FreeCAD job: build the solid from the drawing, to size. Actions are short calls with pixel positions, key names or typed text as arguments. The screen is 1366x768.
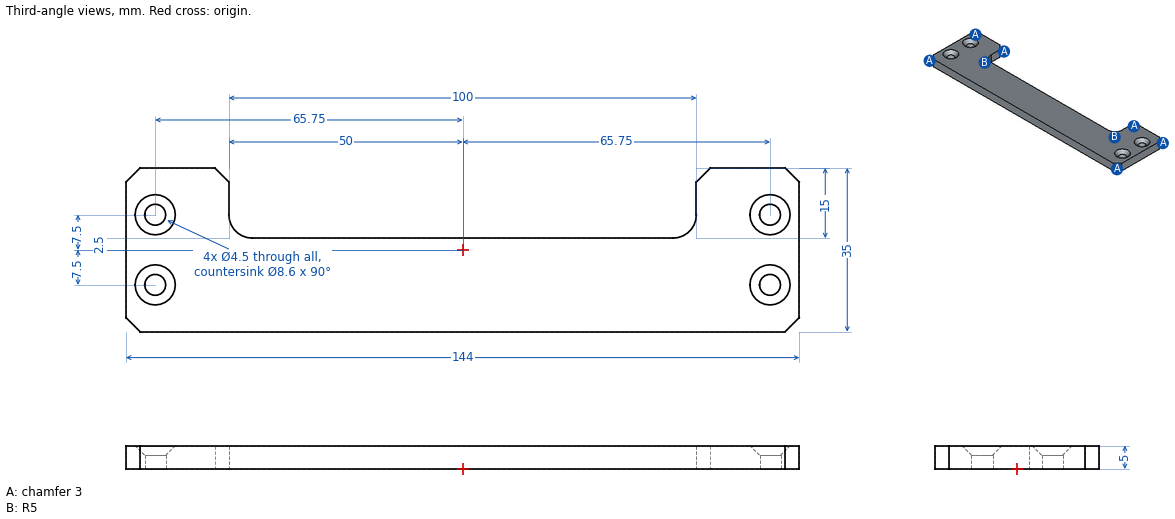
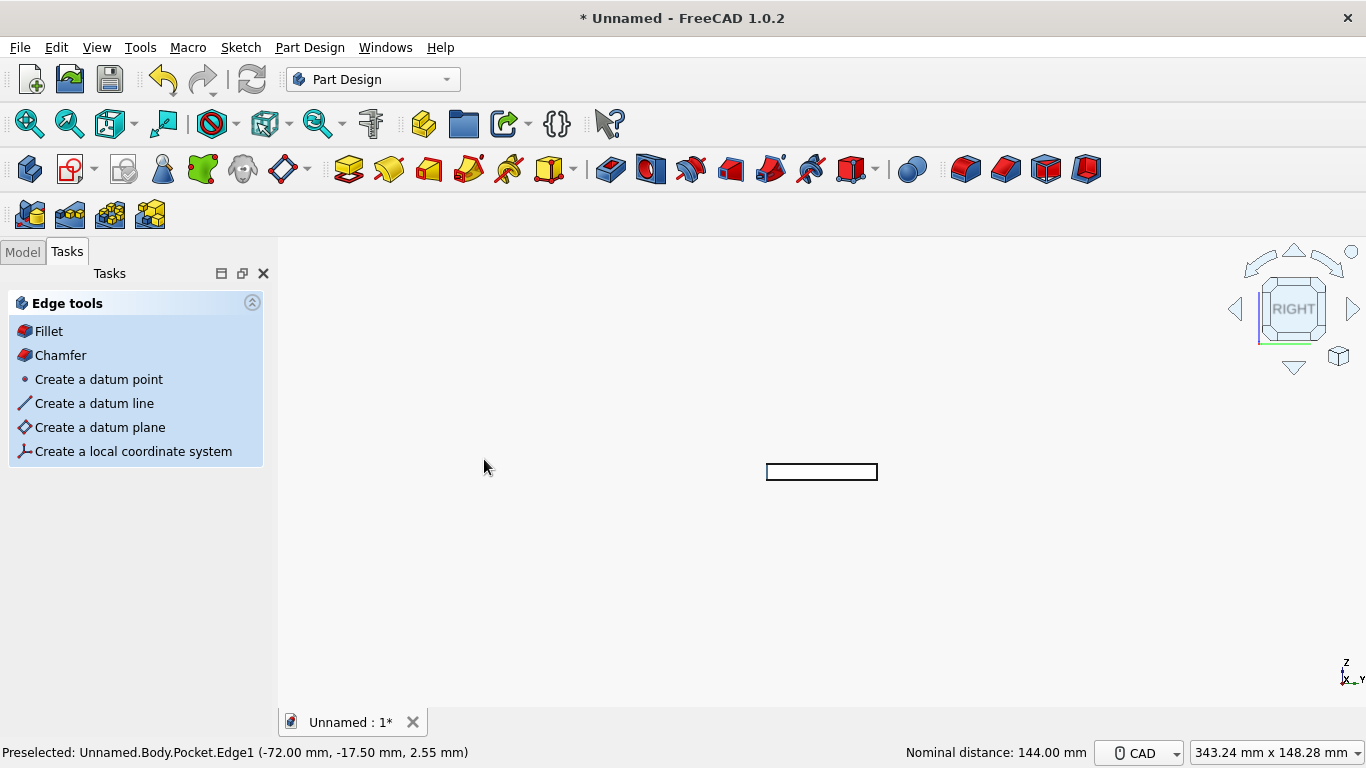
click(877, 471, ctrl)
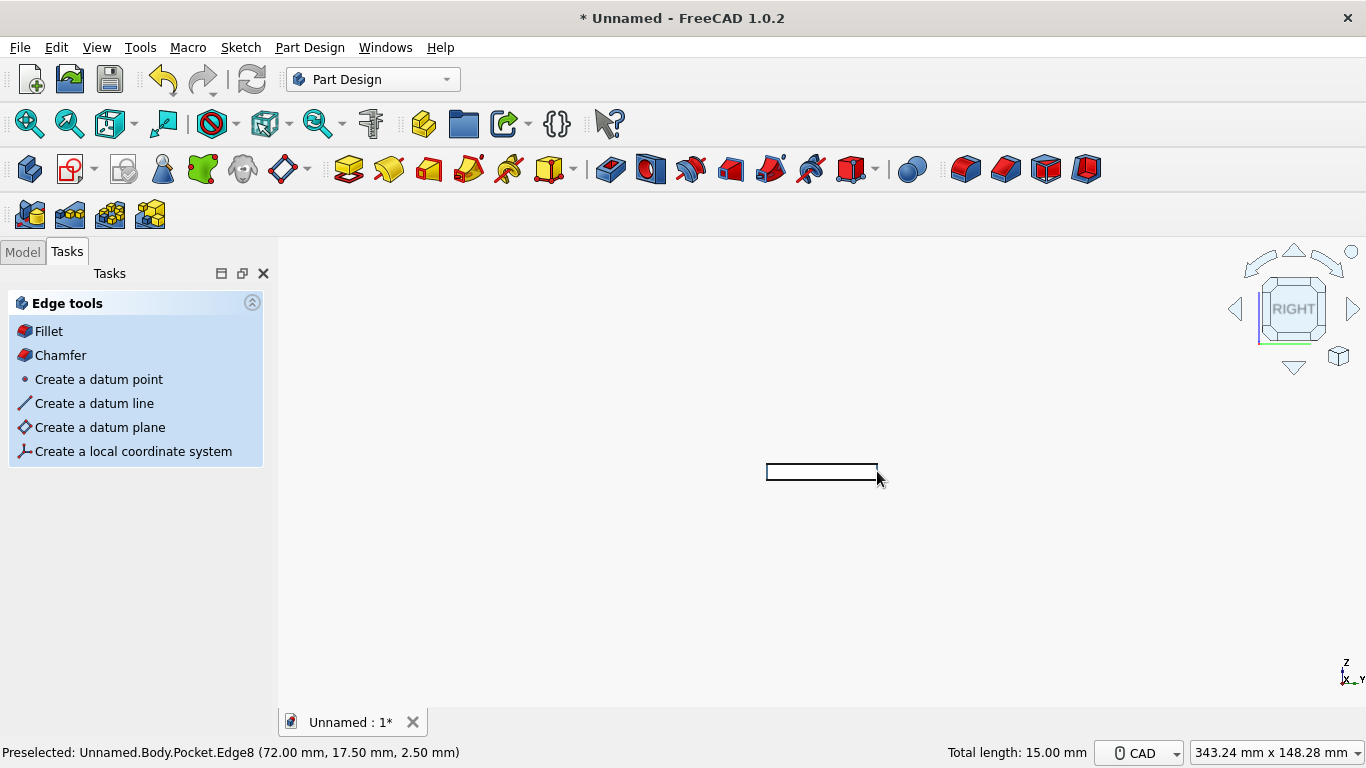
scroll(877, 471, up, 5)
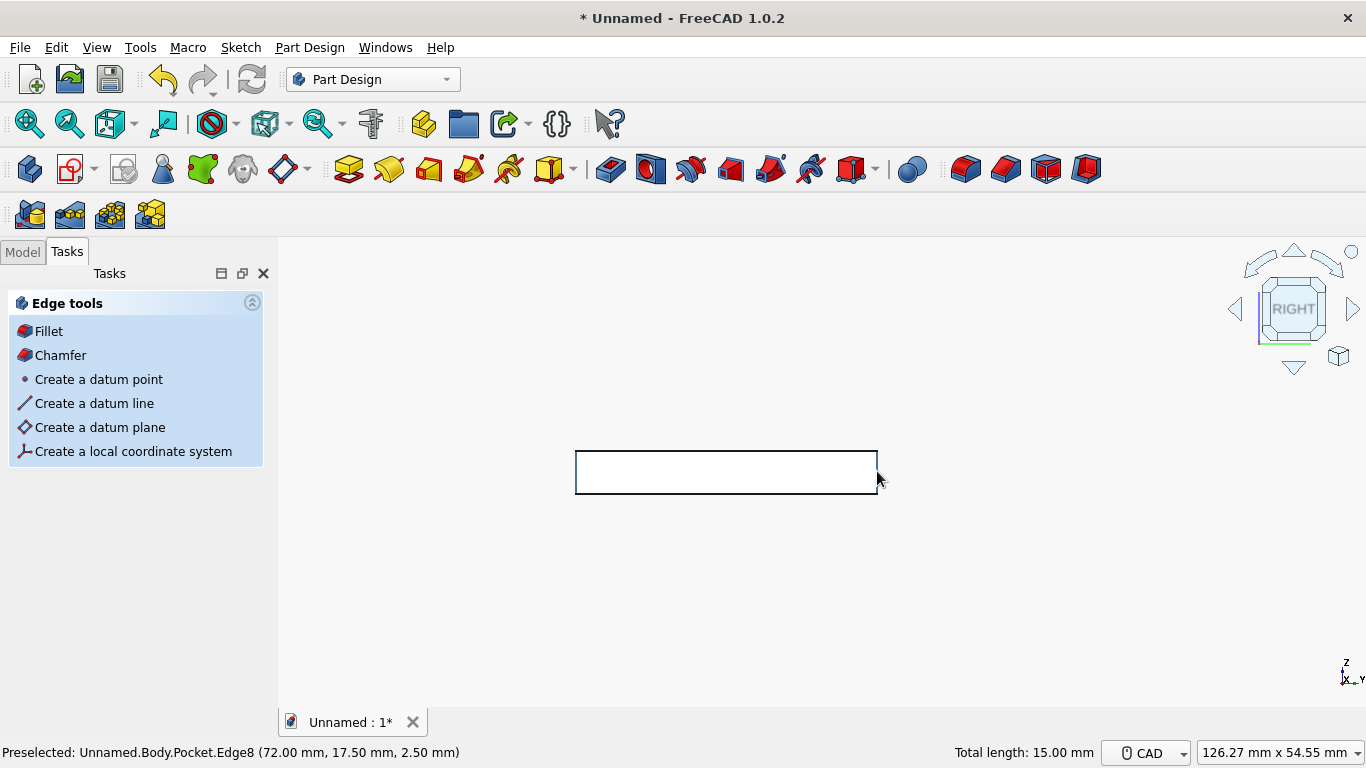
key(v)
key(f)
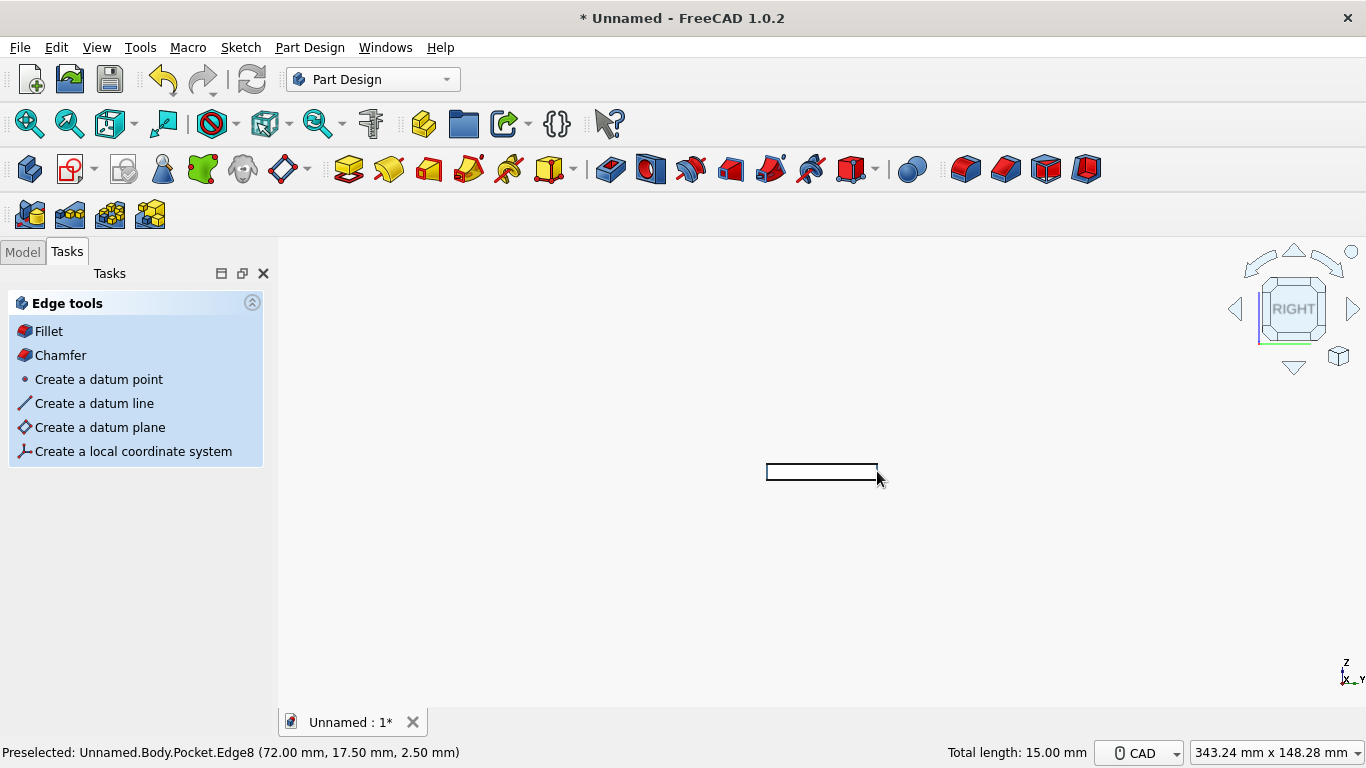
key(5)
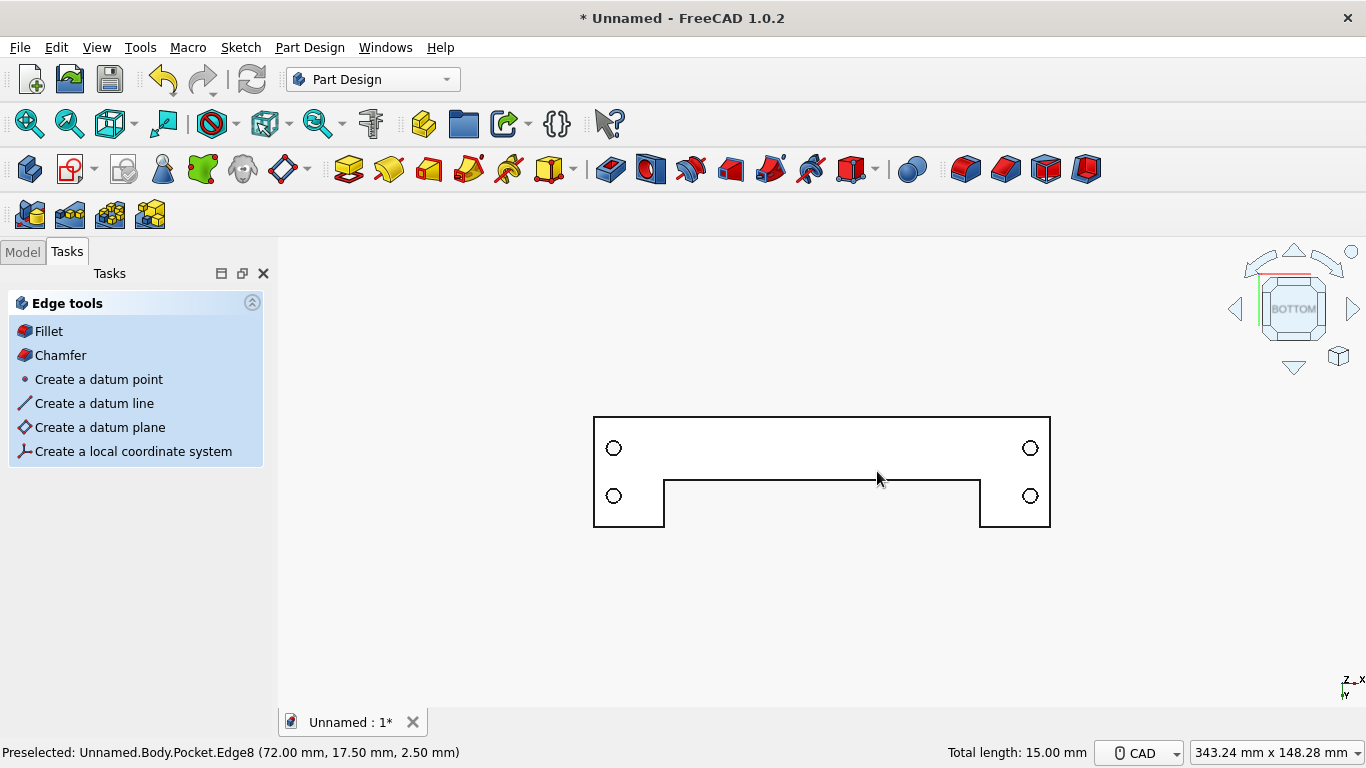
click(30, 124)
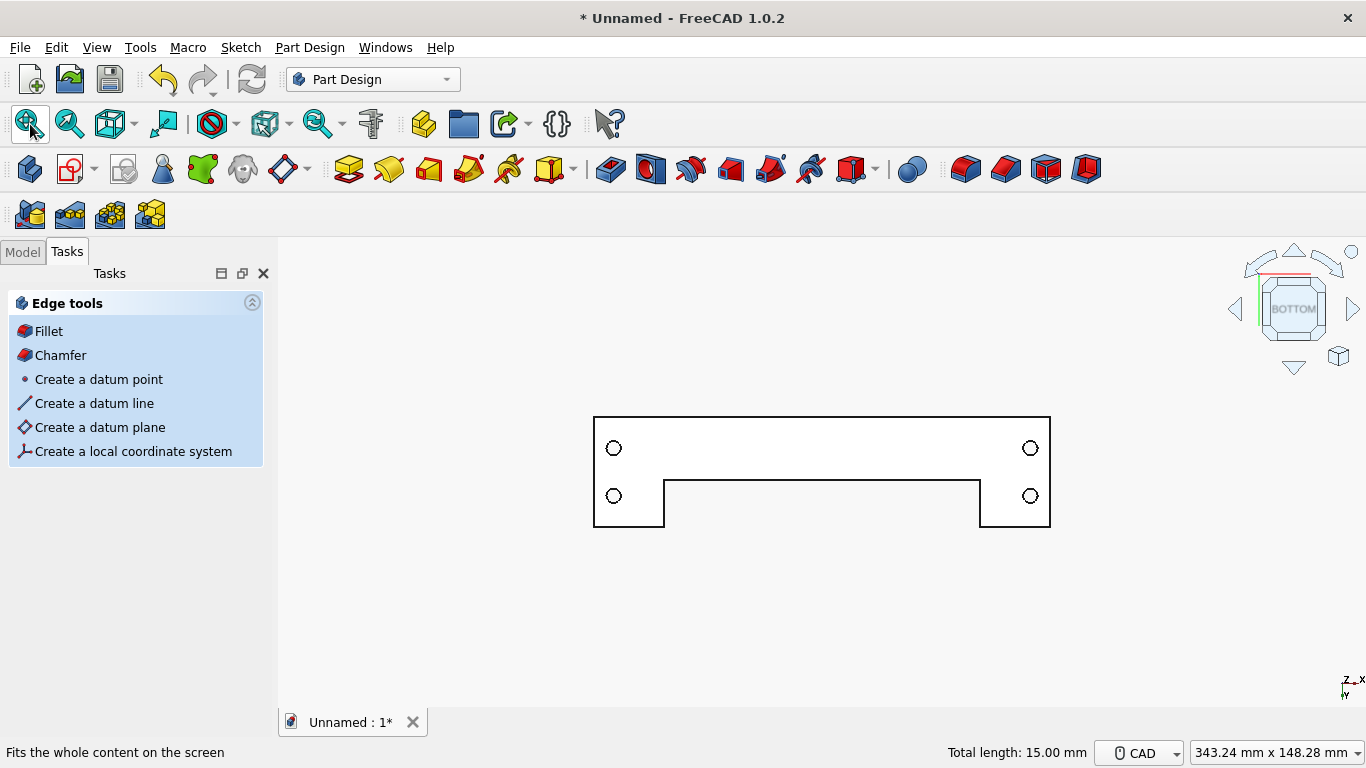
scroll(664, 526, up, 5)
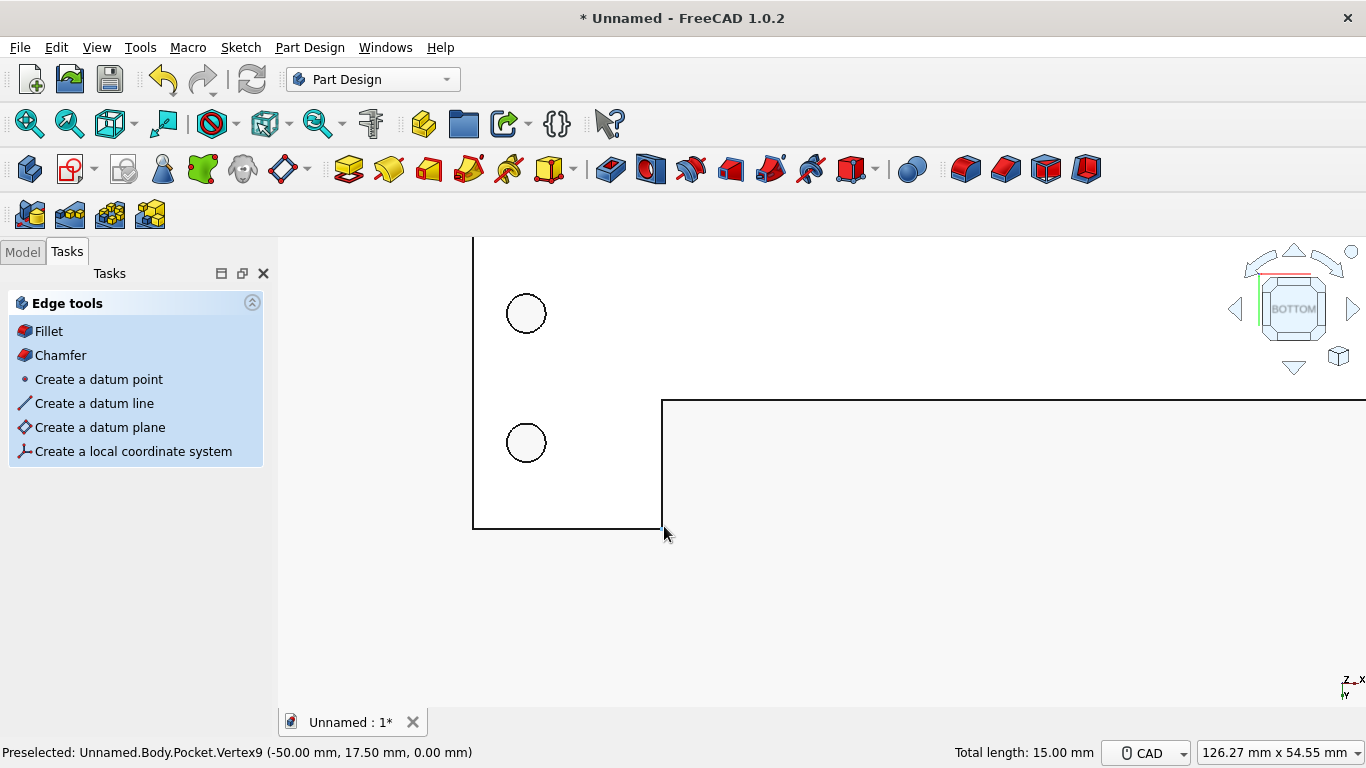
key(v)
key(f)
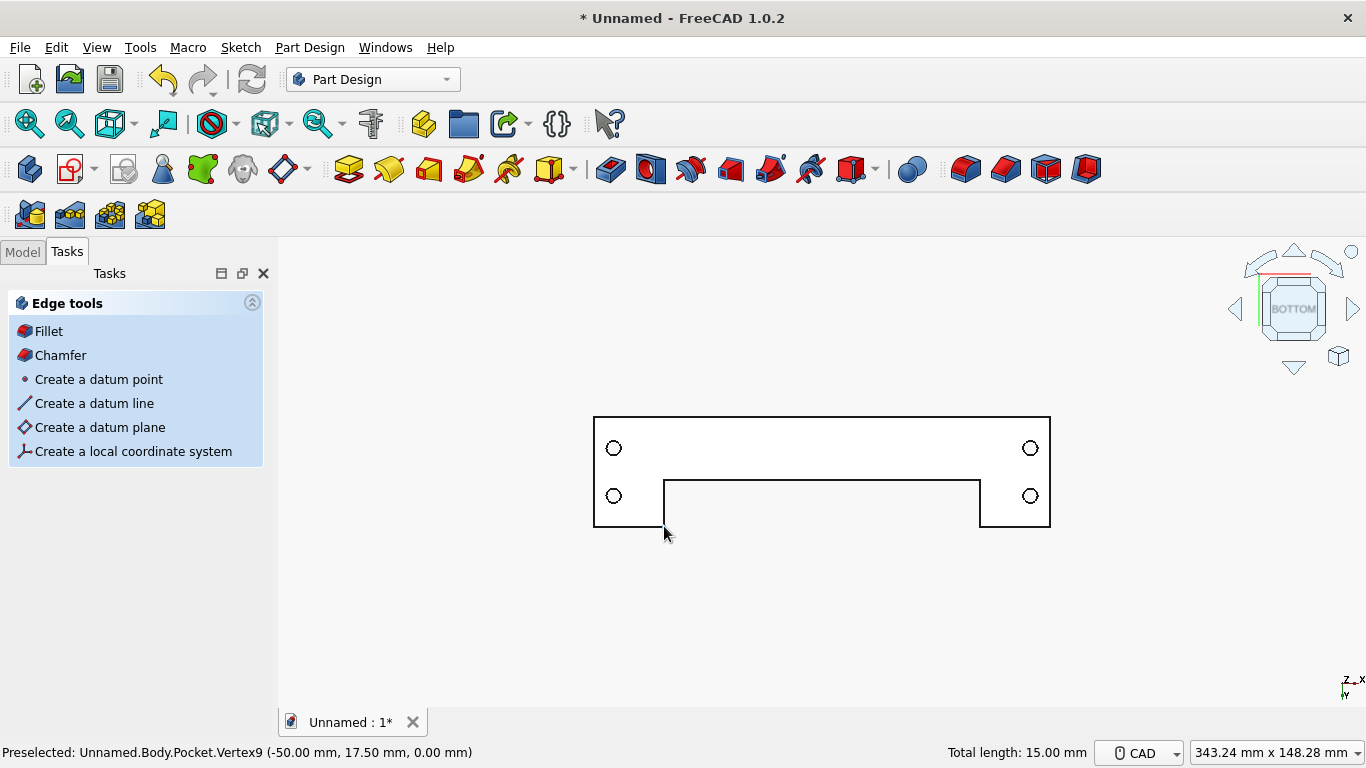
key(4)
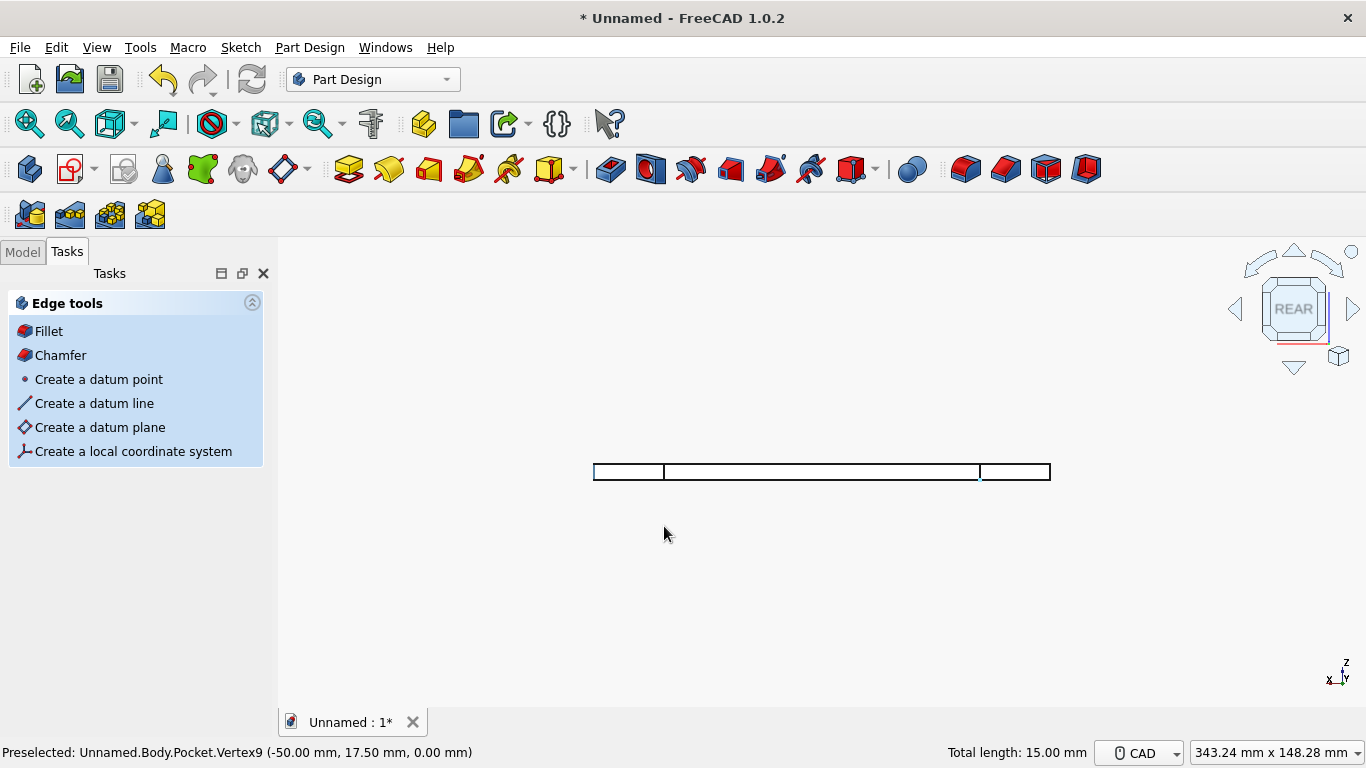
key(v)
key(f)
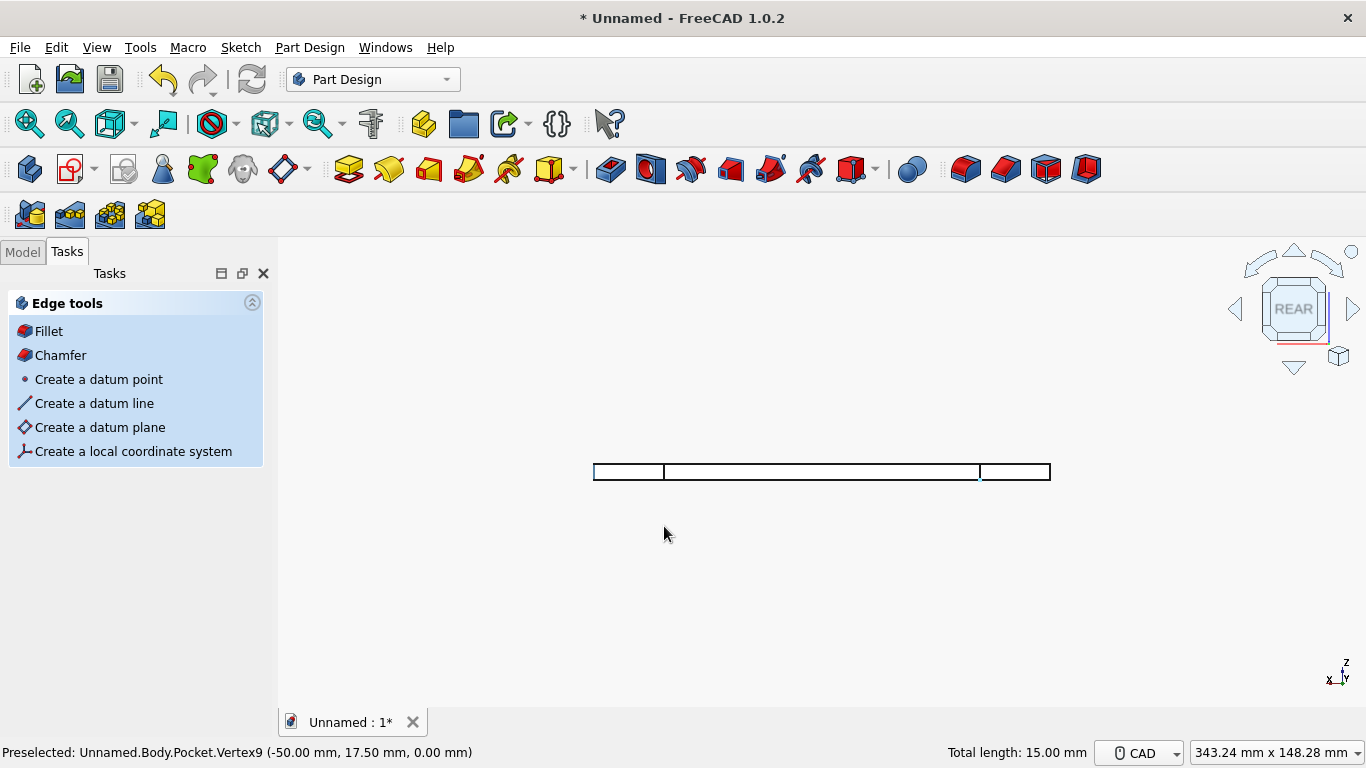
click(980, 471, ctrl)